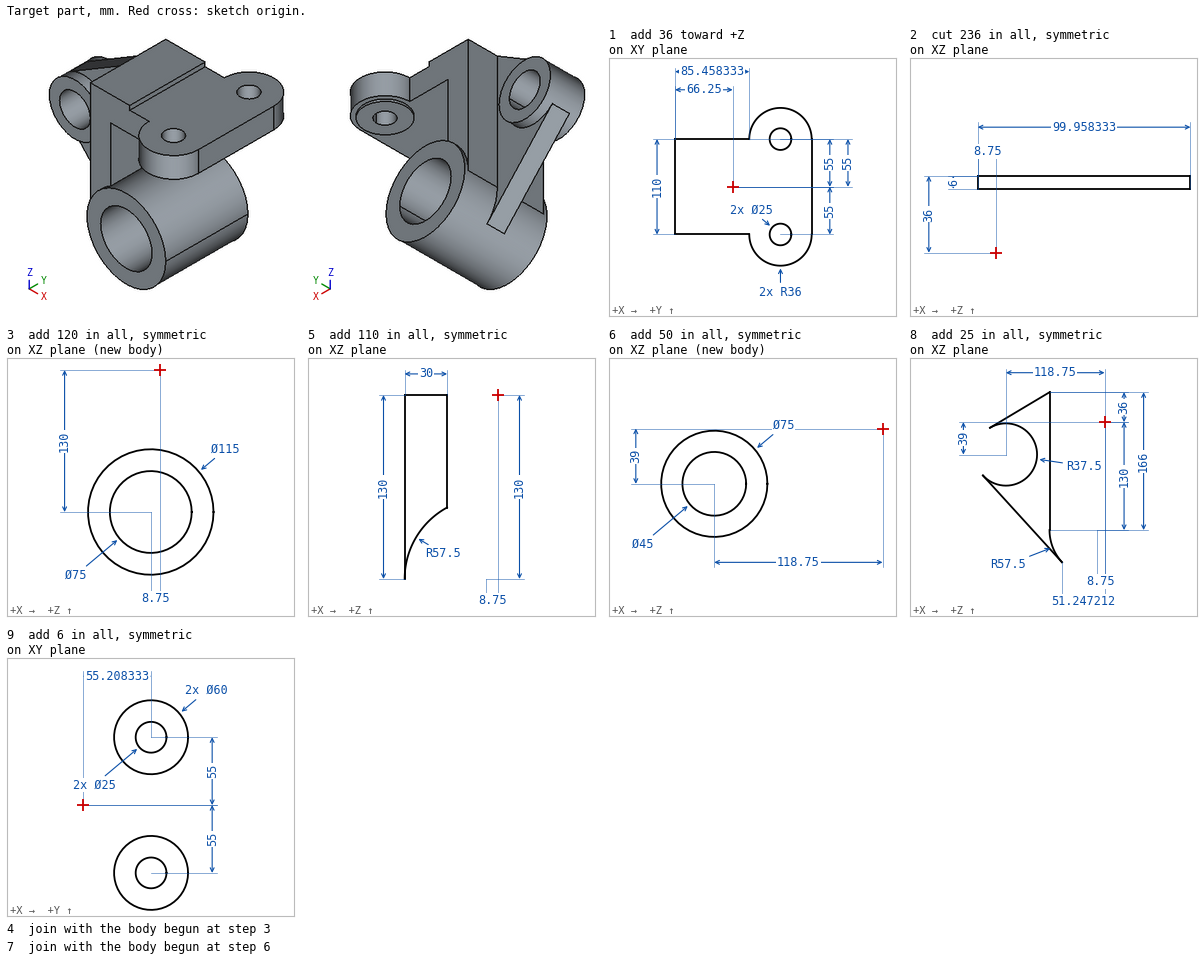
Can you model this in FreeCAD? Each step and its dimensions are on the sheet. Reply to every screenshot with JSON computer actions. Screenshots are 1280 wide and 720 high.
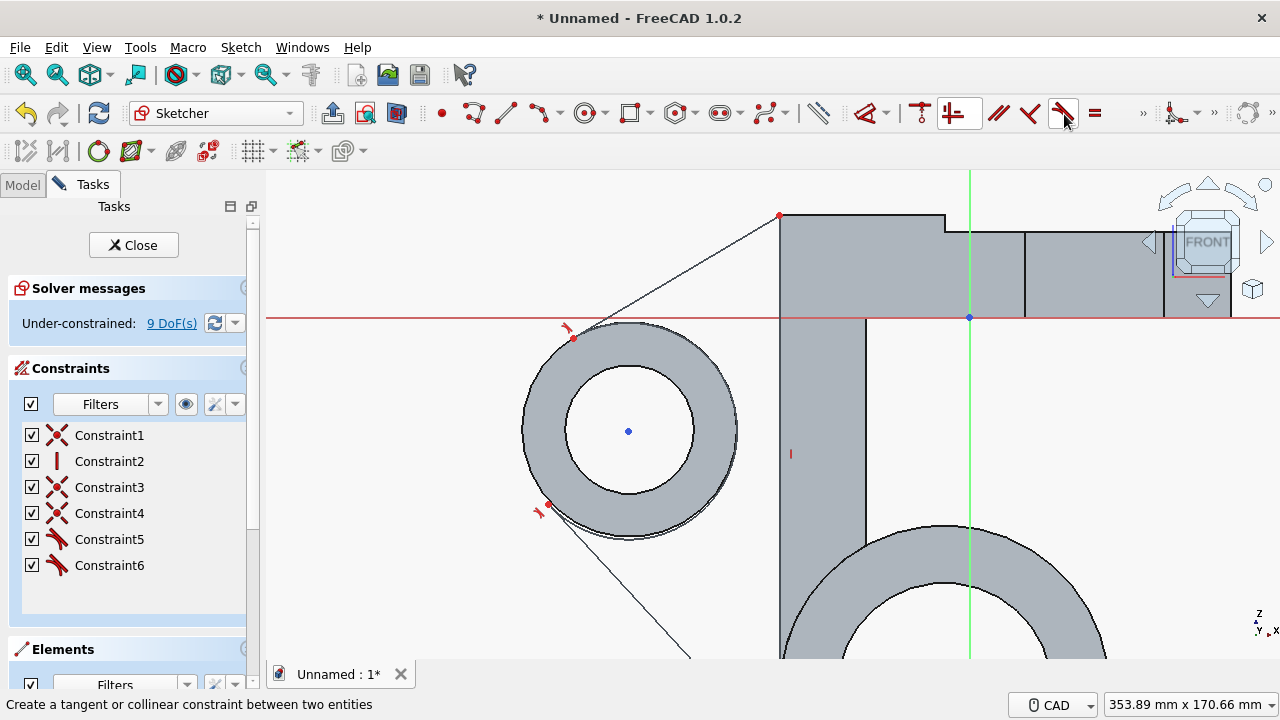
{"action": "left_click", "coordinate": [866, 114]}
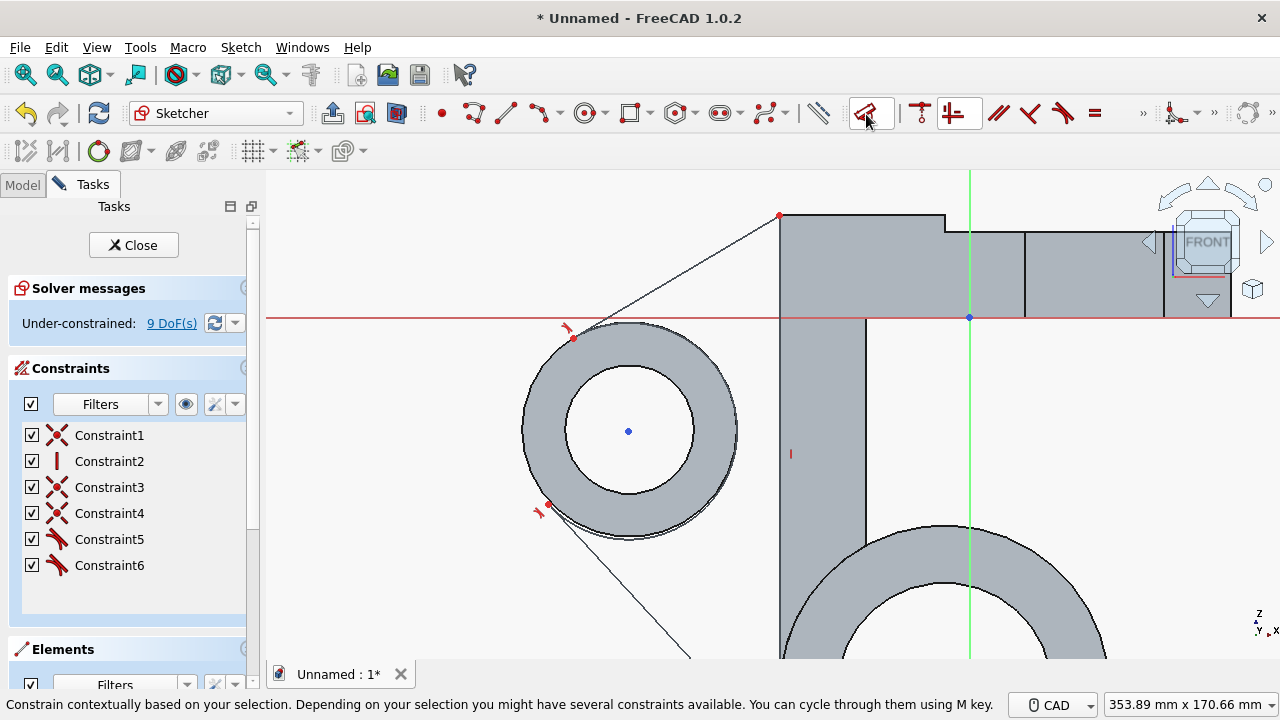
{"action": "left_click", "coordinate": [683, 525]}
{"action": "left_click", "coordinate": [699, 553]}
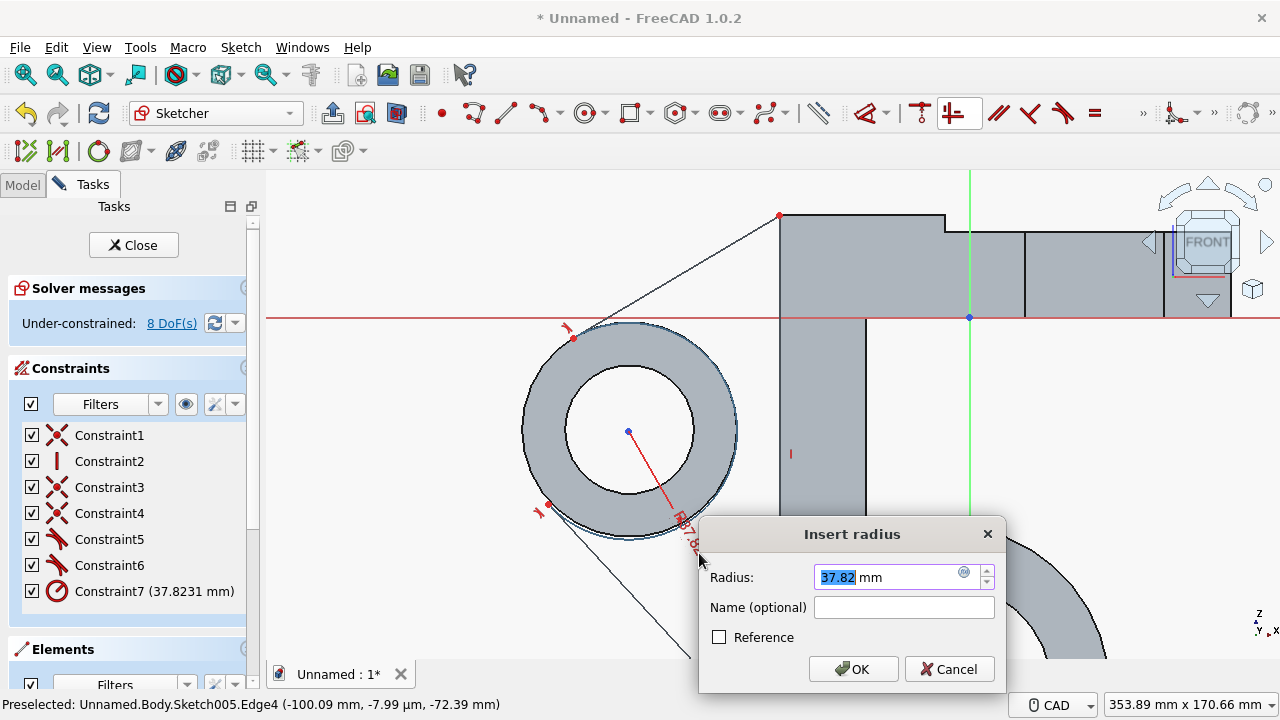
{"action": "type", "text": "37.5"}
{"action": "key", "text": "Return"}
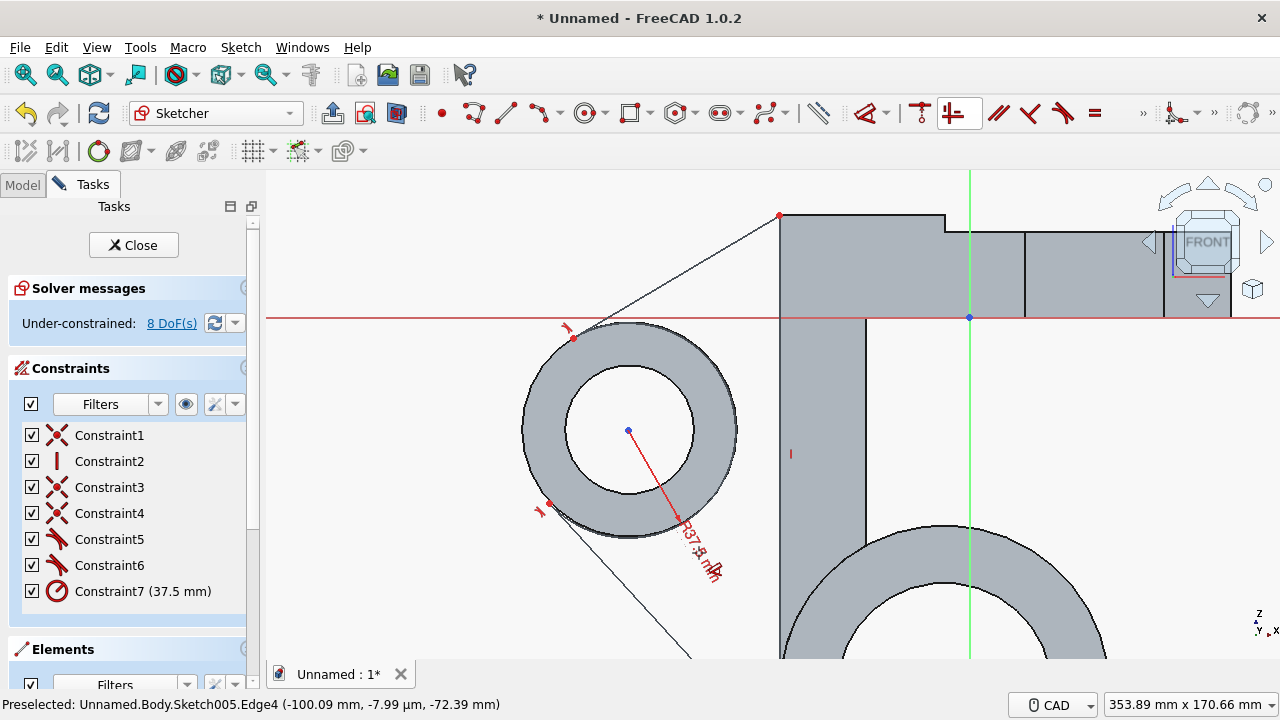
{"action": "scroll", "coordinate": [637, 301], "scroll_direction": "down", "scroll_amount": 3}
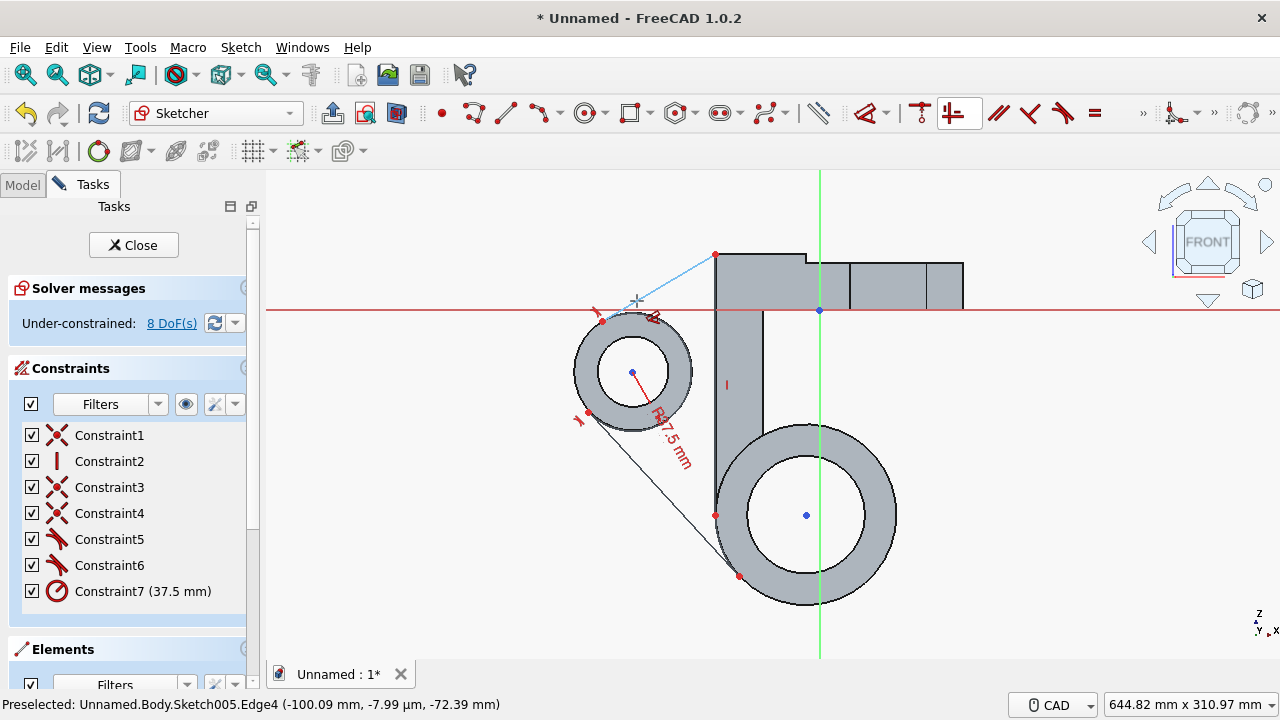
{"action": "left_click", "coordinate": [718, 535]}
{"action": "left_click", "coordinate": [687, 542]}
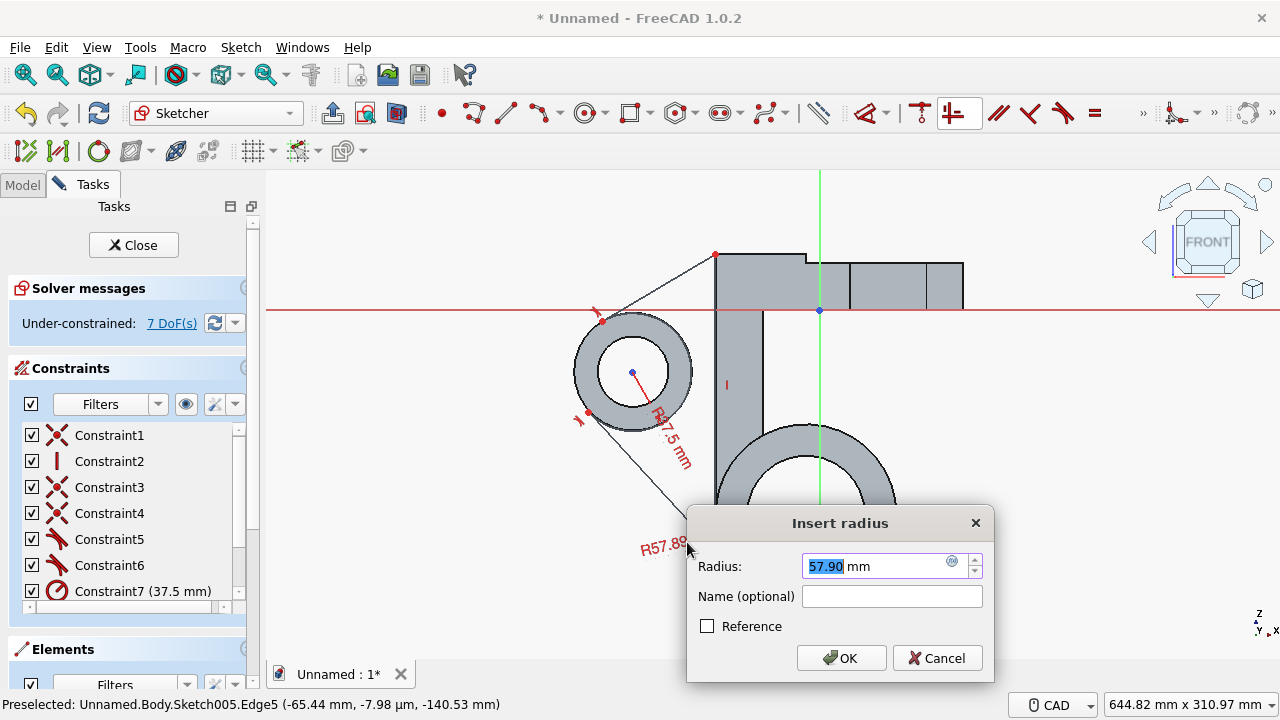
{"action": "type", "text": "57.5"}
{"action": "key", "text": "Return"}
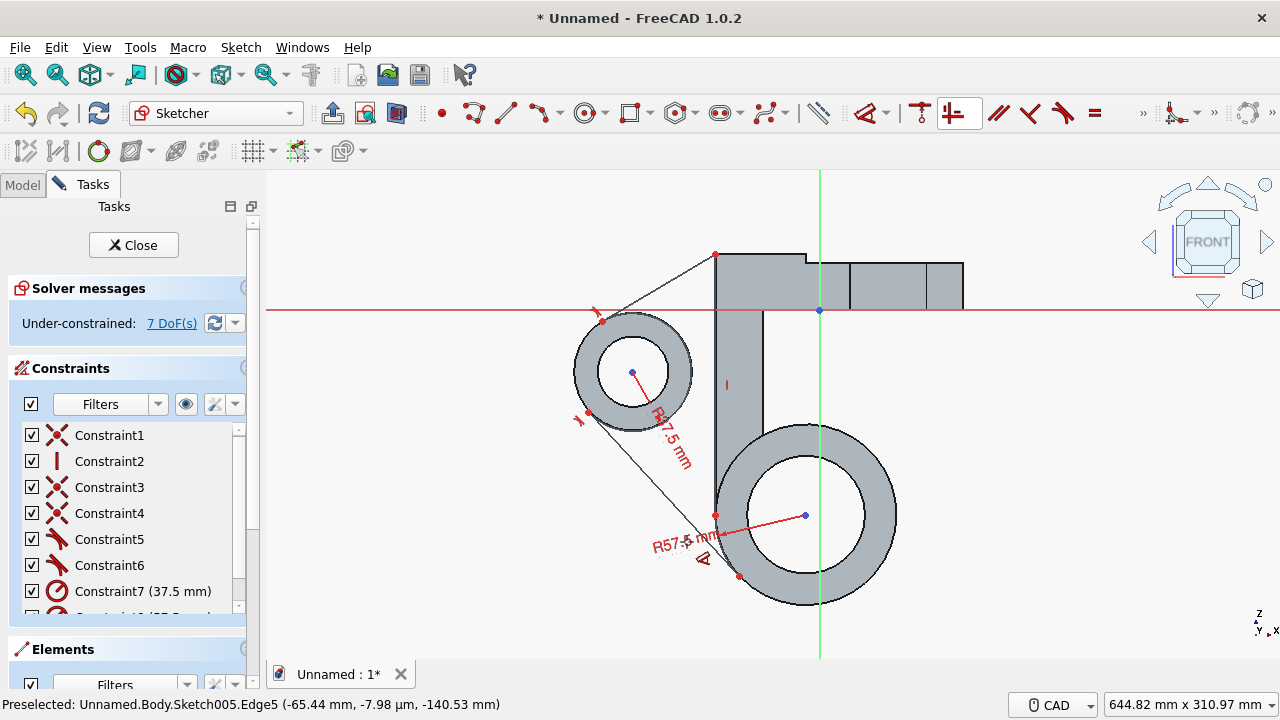
{"action": "left_click", "coordinate": [715, 333]}
{"action": "left_click", "coordinate": [749, 385]}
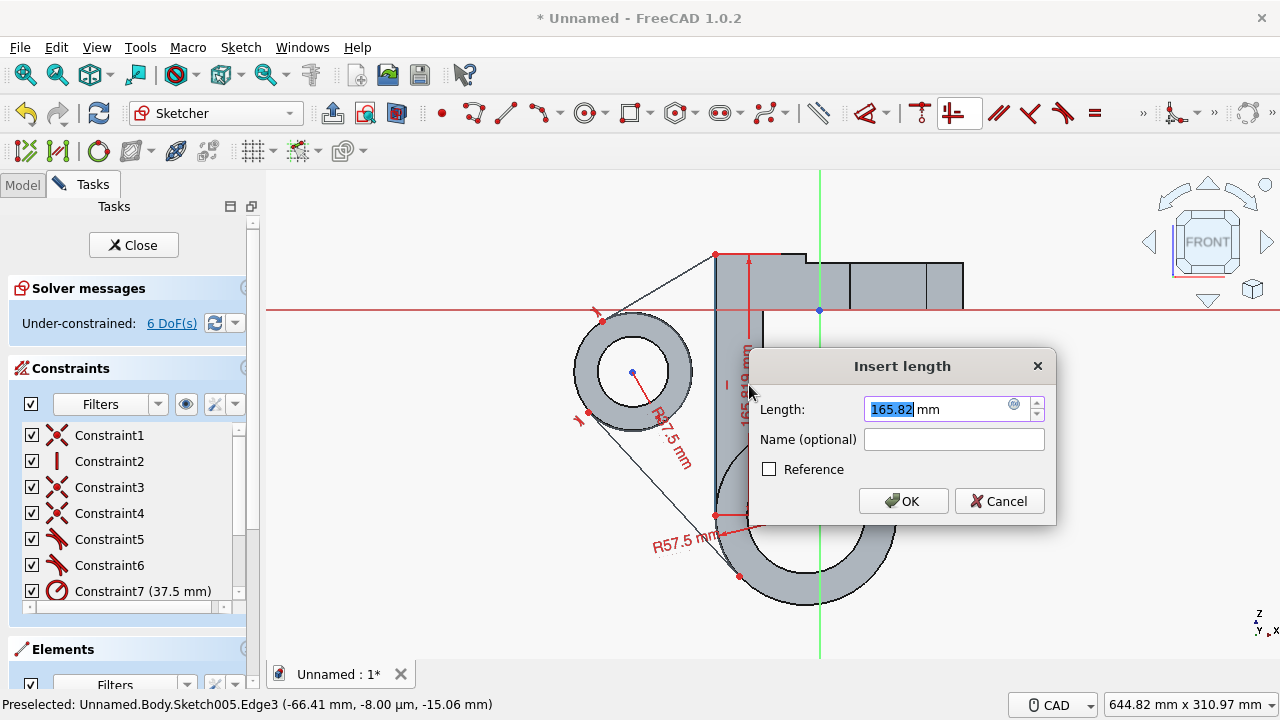
{"action": "type", "text": "166"}
{"action": "key", "text": "Return"}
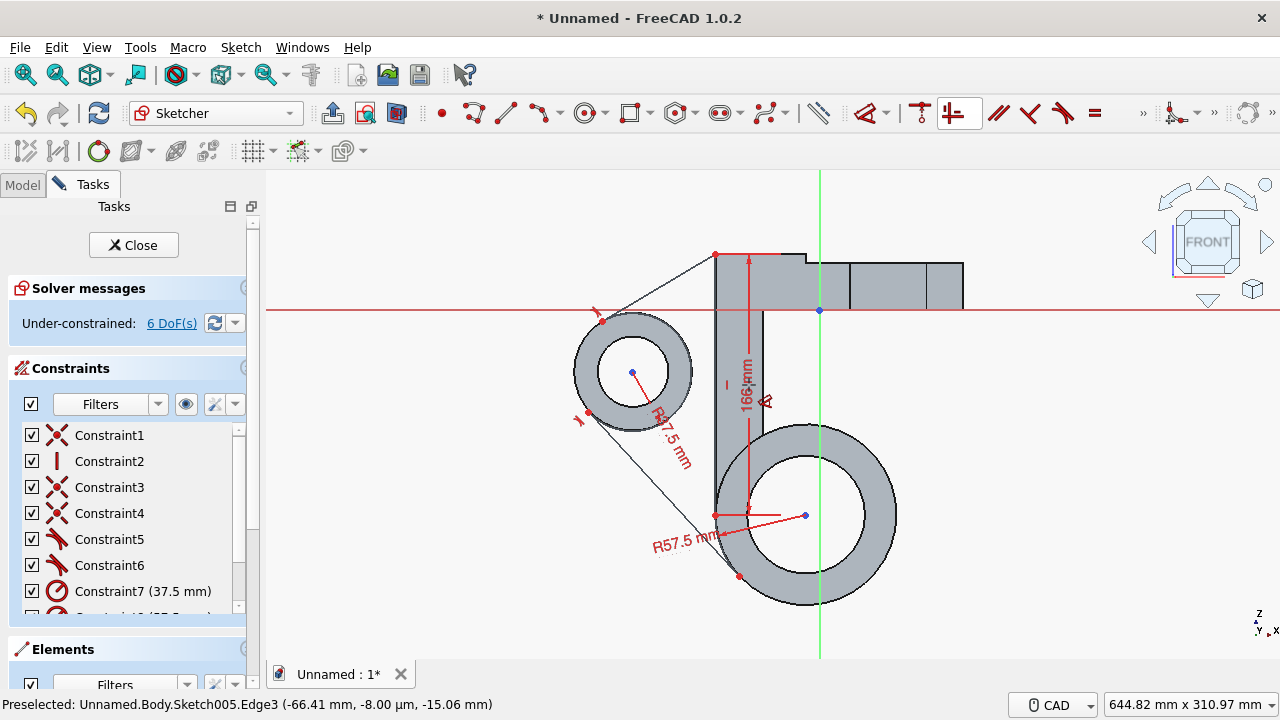
{"action": "left_click", "coordinate": [715, 254]}
{"action": "left_click", "coordinate": [854, 282]}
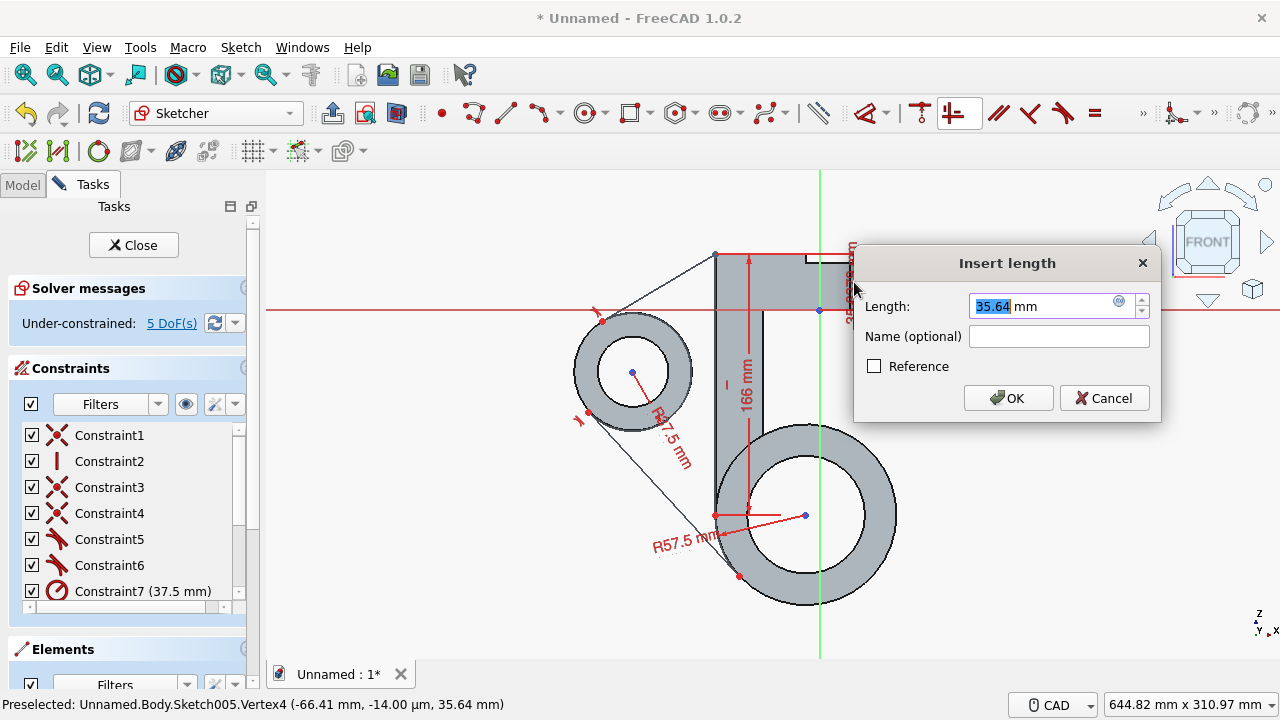
{"action": "type", "text": "36"}
{"action": "key", "text": "Return"}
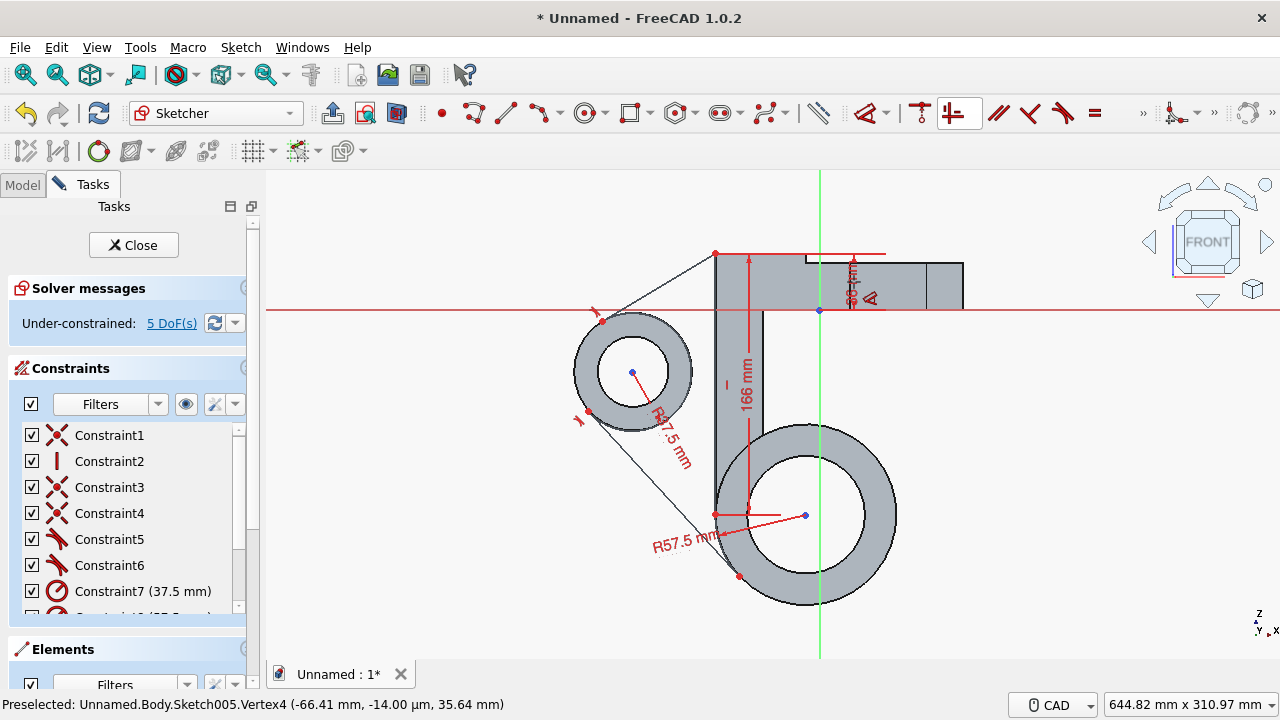
{"action": "left_click", "coordinate": [632, 372]}
{"action": "left_click", "coordinate": [854, 341]}